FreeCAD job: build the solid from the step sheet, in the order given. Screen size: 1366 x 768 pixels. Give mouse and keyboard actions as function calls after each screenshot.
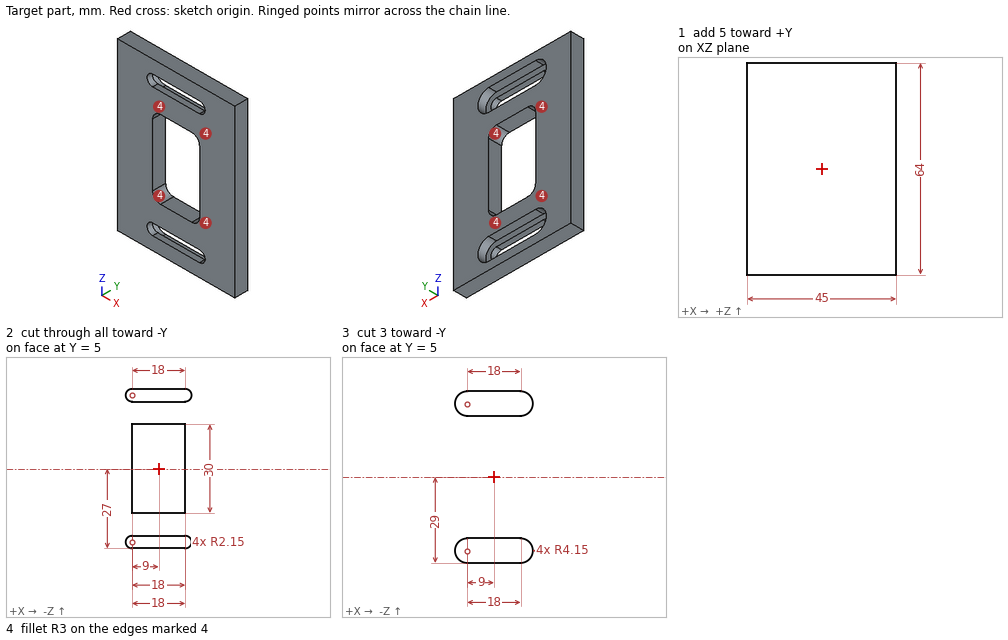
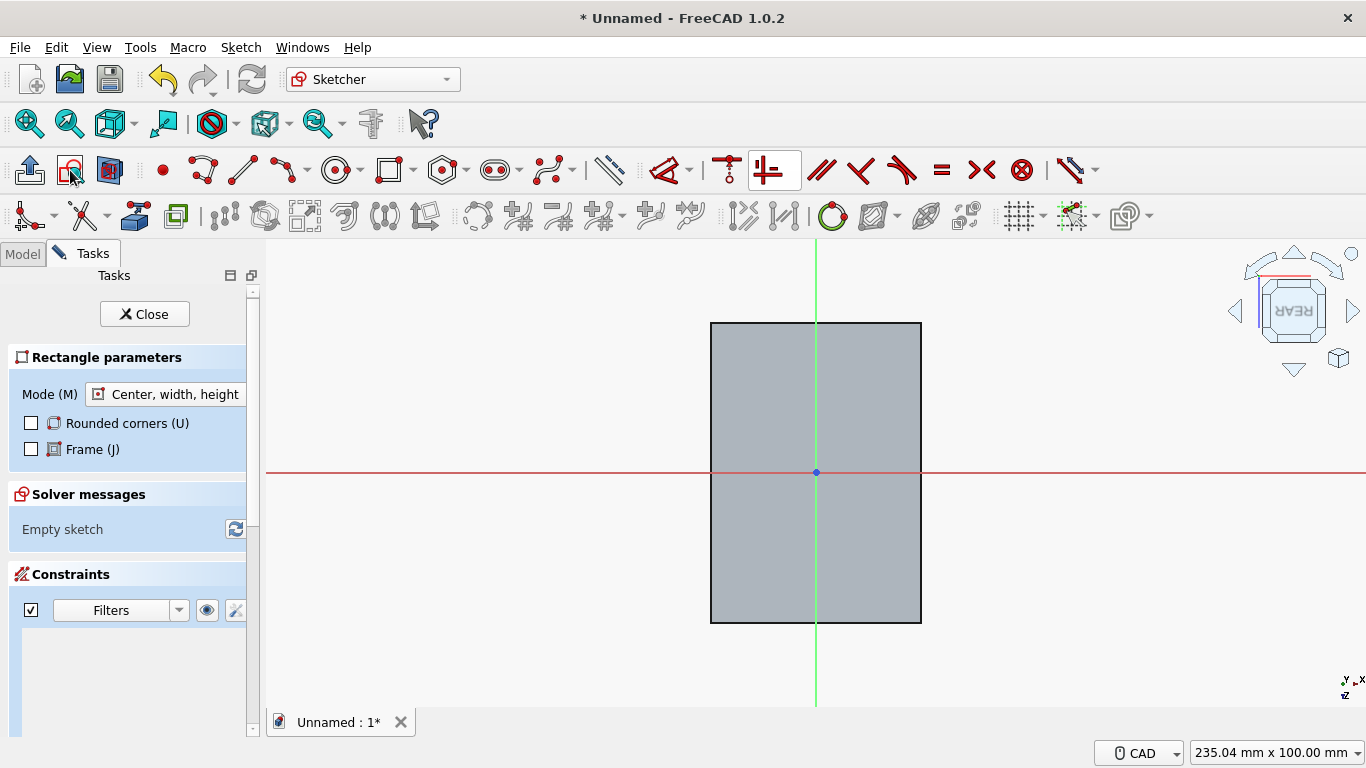
click(816, 473)
click(858, 403)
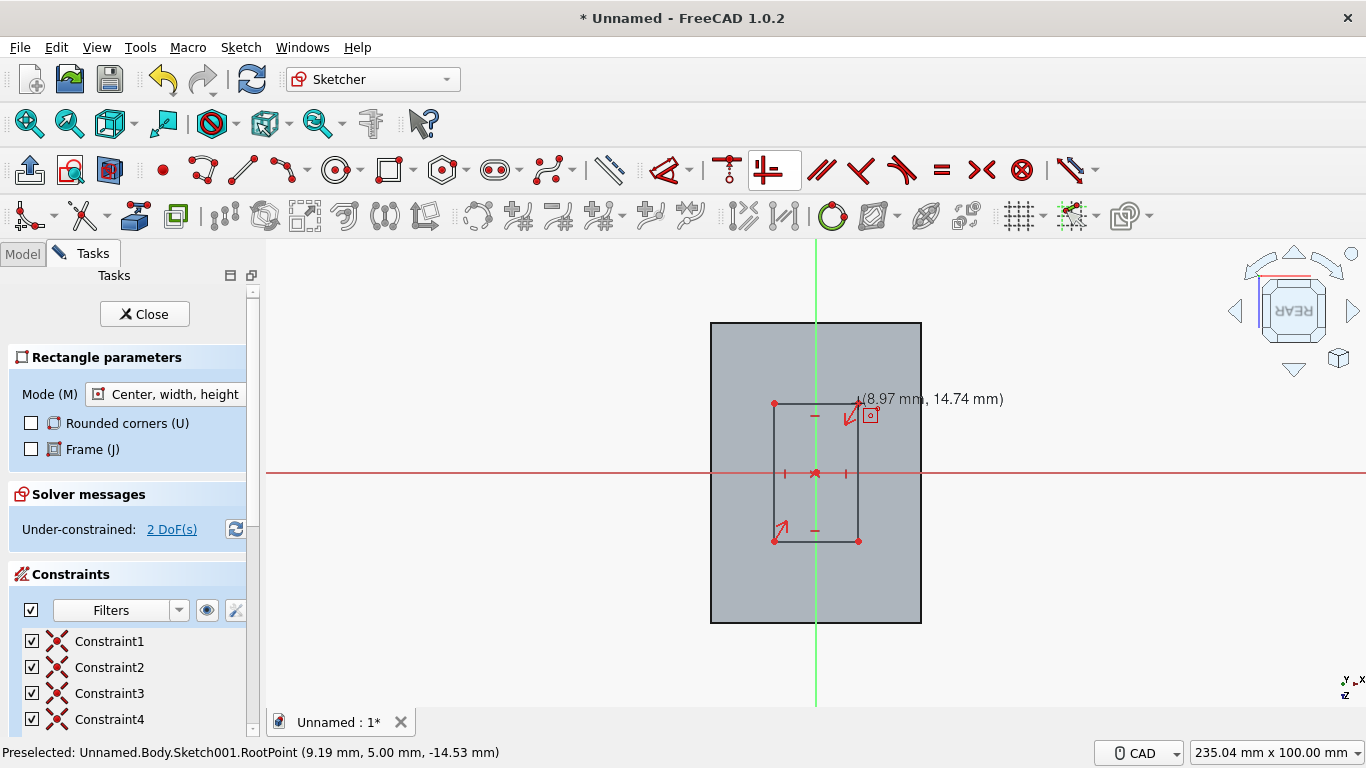
click(496, 170)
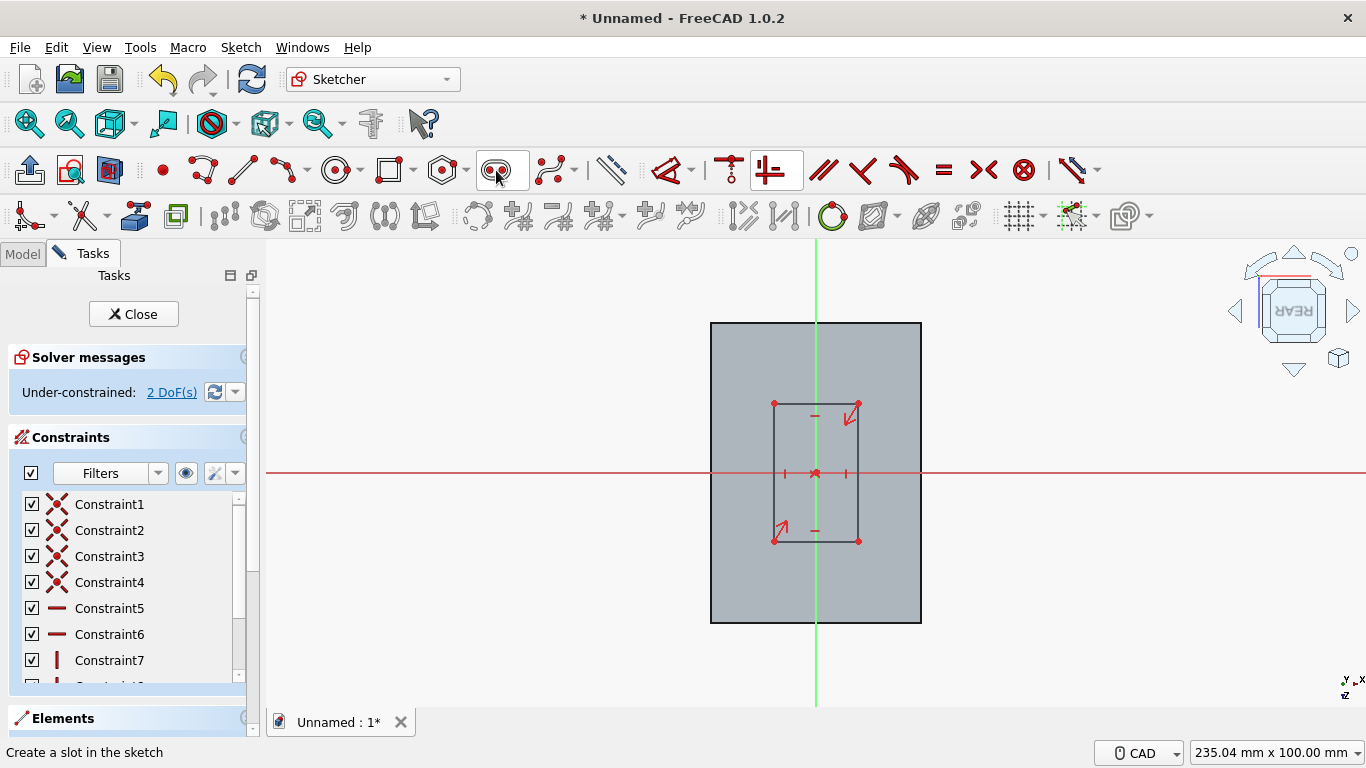
scroll(774, 589, up, 5)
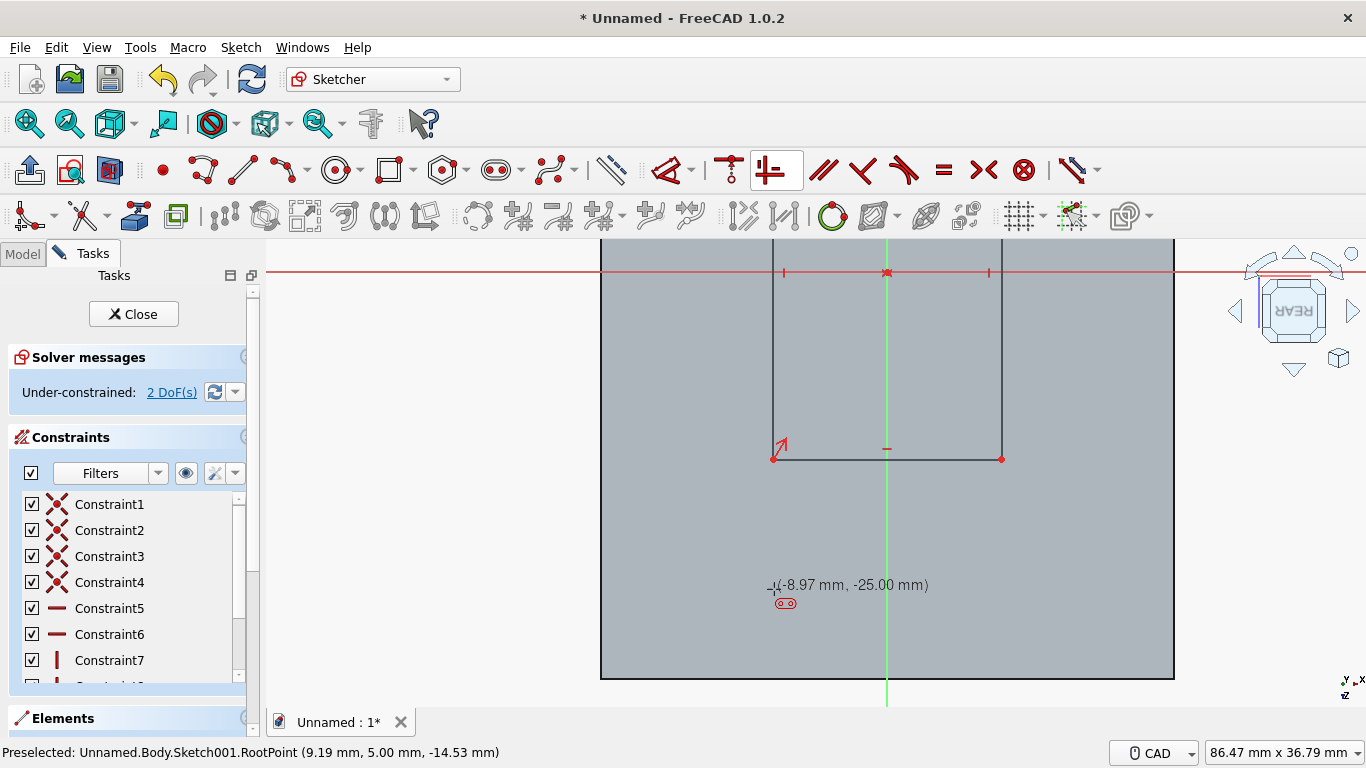
click(773, 589)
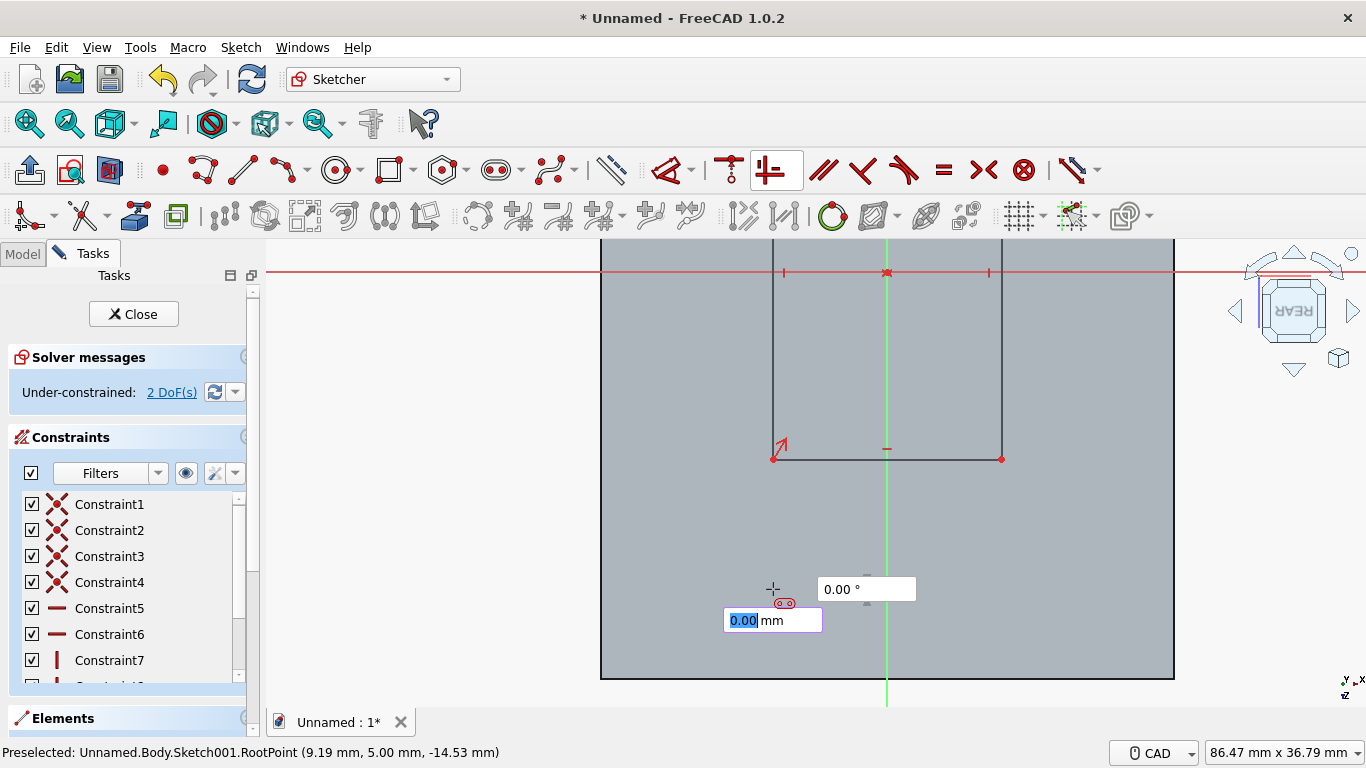
click(1002, 589)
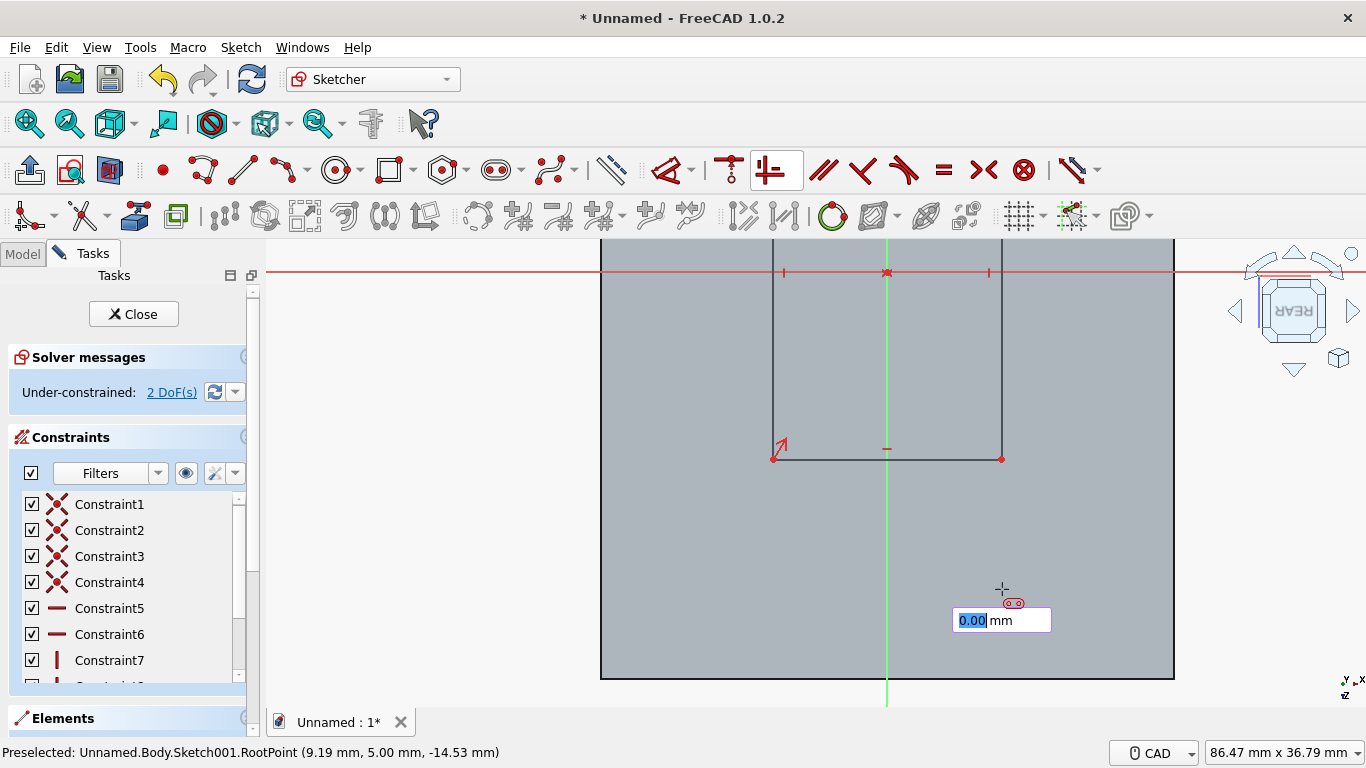
click(922, 561)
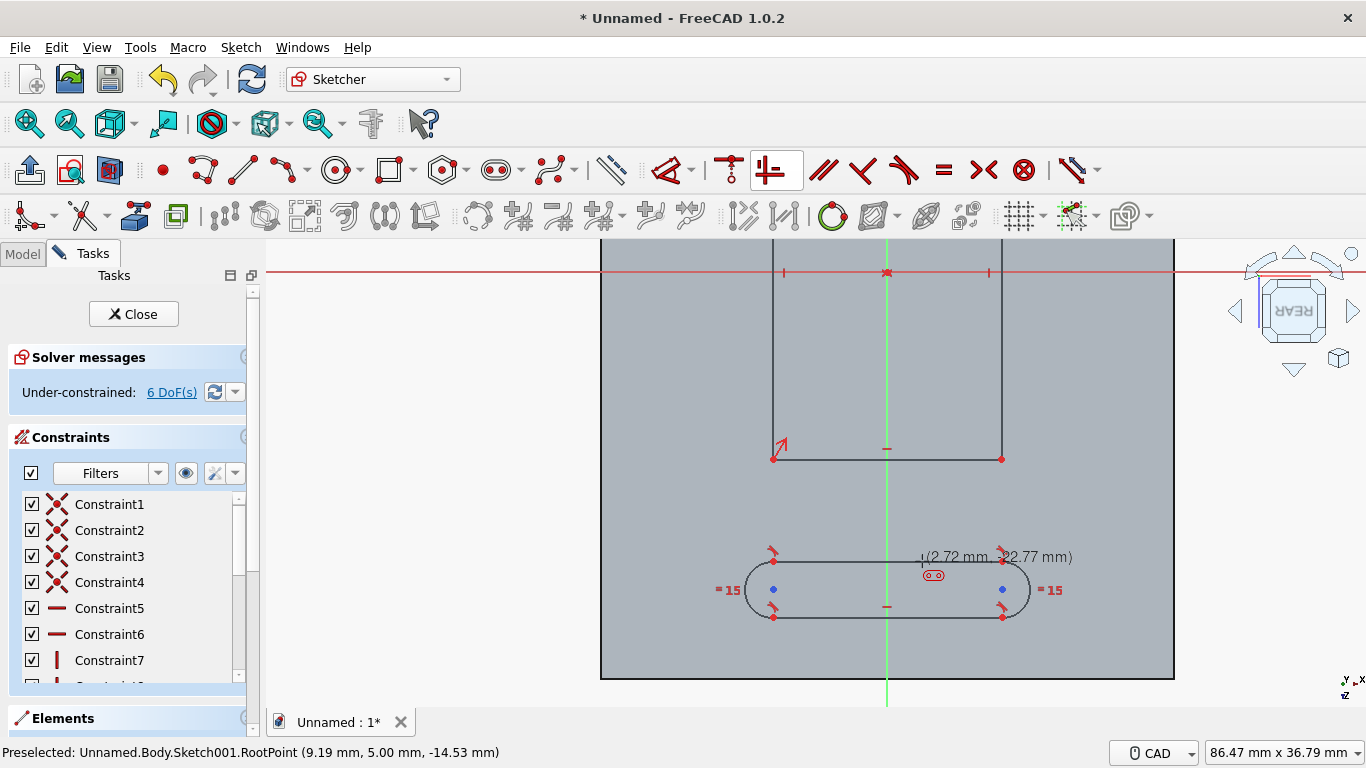
scroll(633, 637, down, 4)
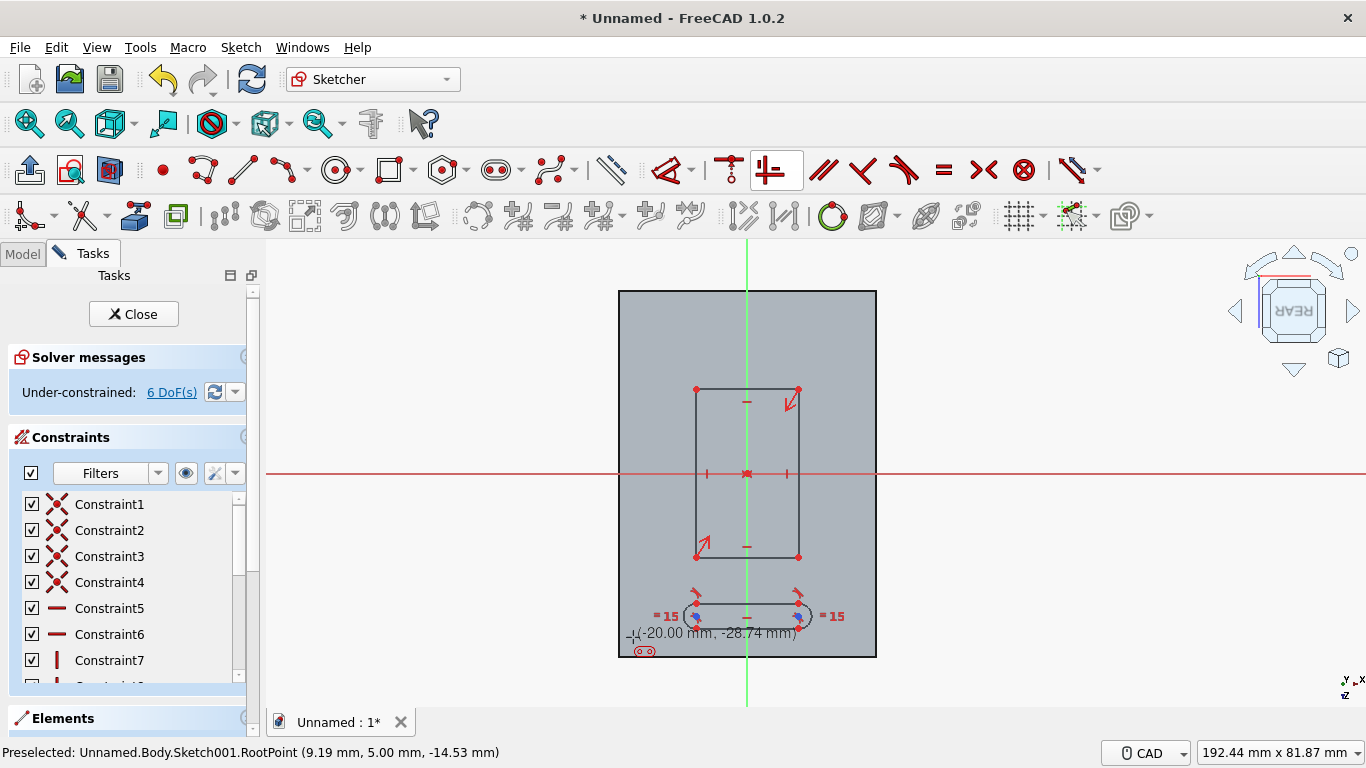
scroll(696, 332, up, 4)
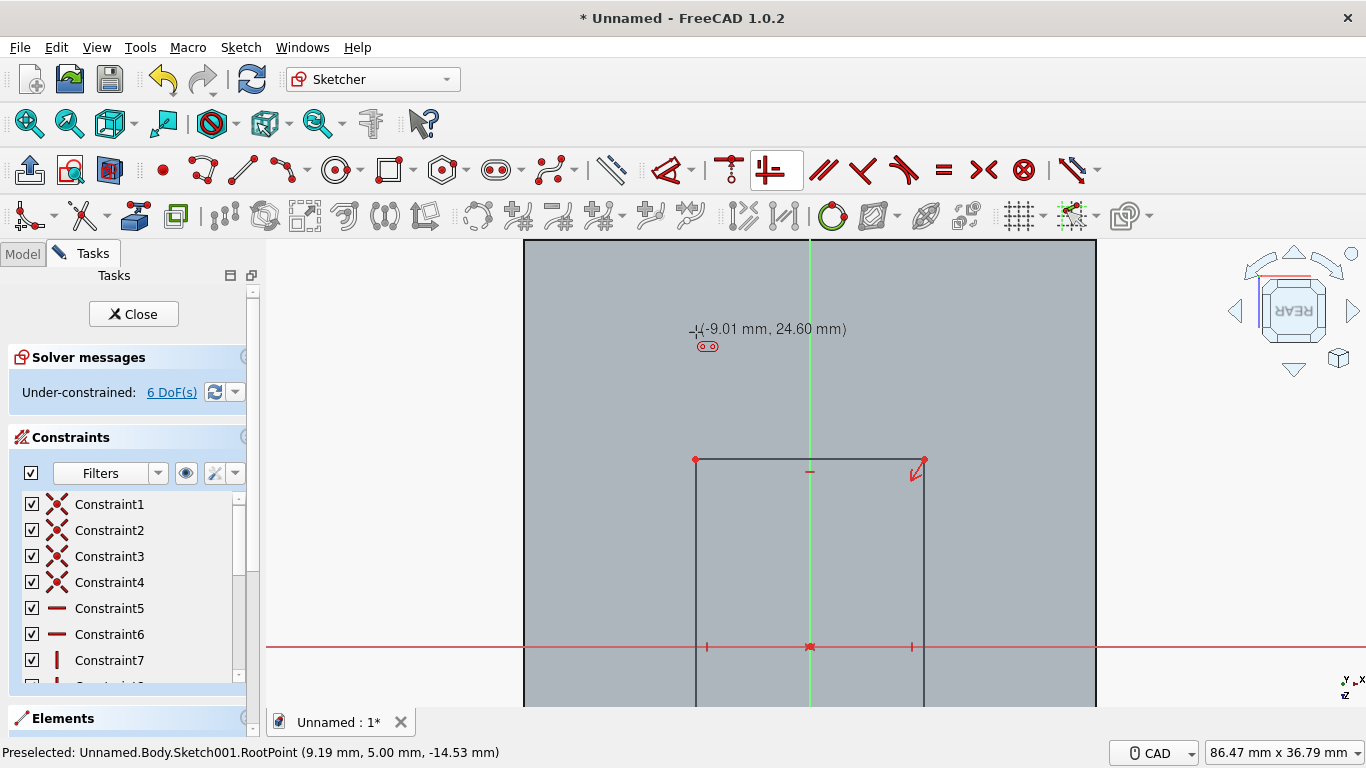
click(696, 331)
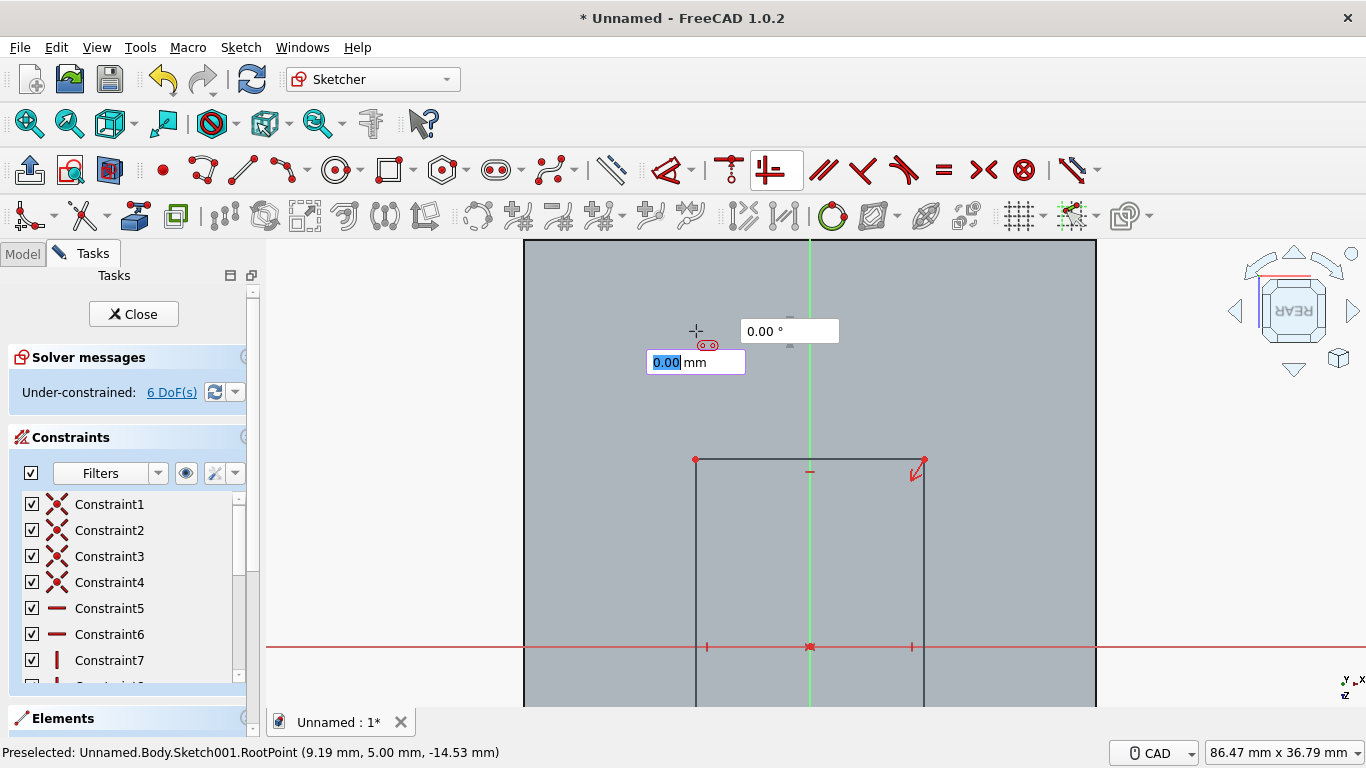
click(925, 331)